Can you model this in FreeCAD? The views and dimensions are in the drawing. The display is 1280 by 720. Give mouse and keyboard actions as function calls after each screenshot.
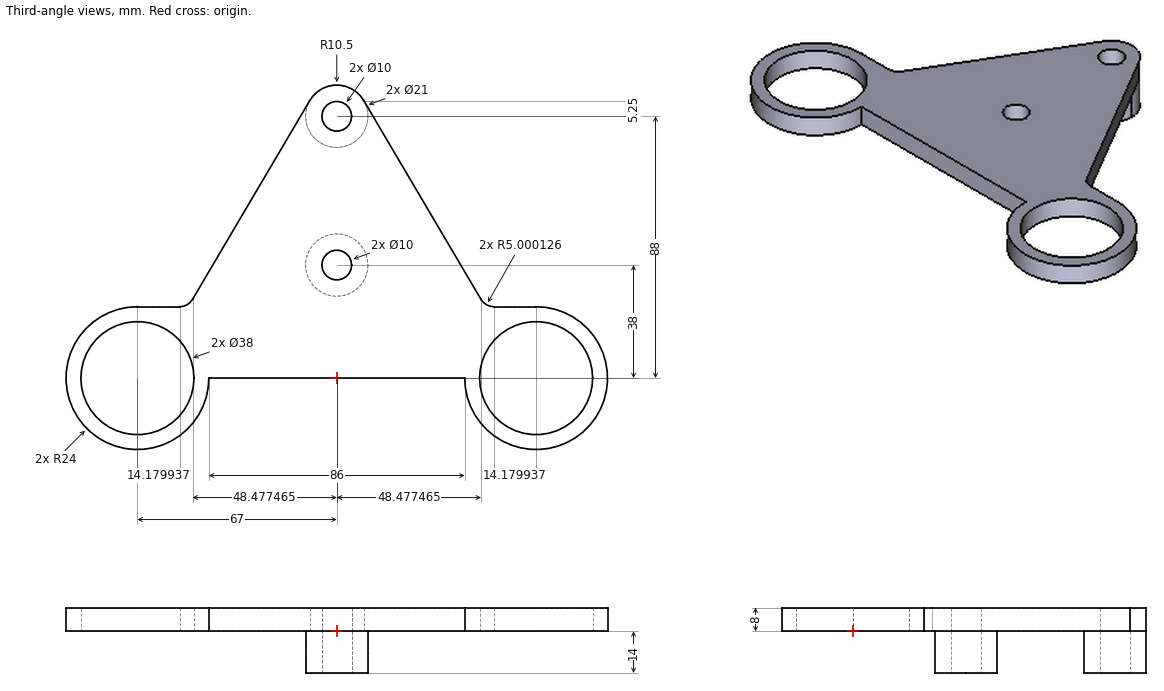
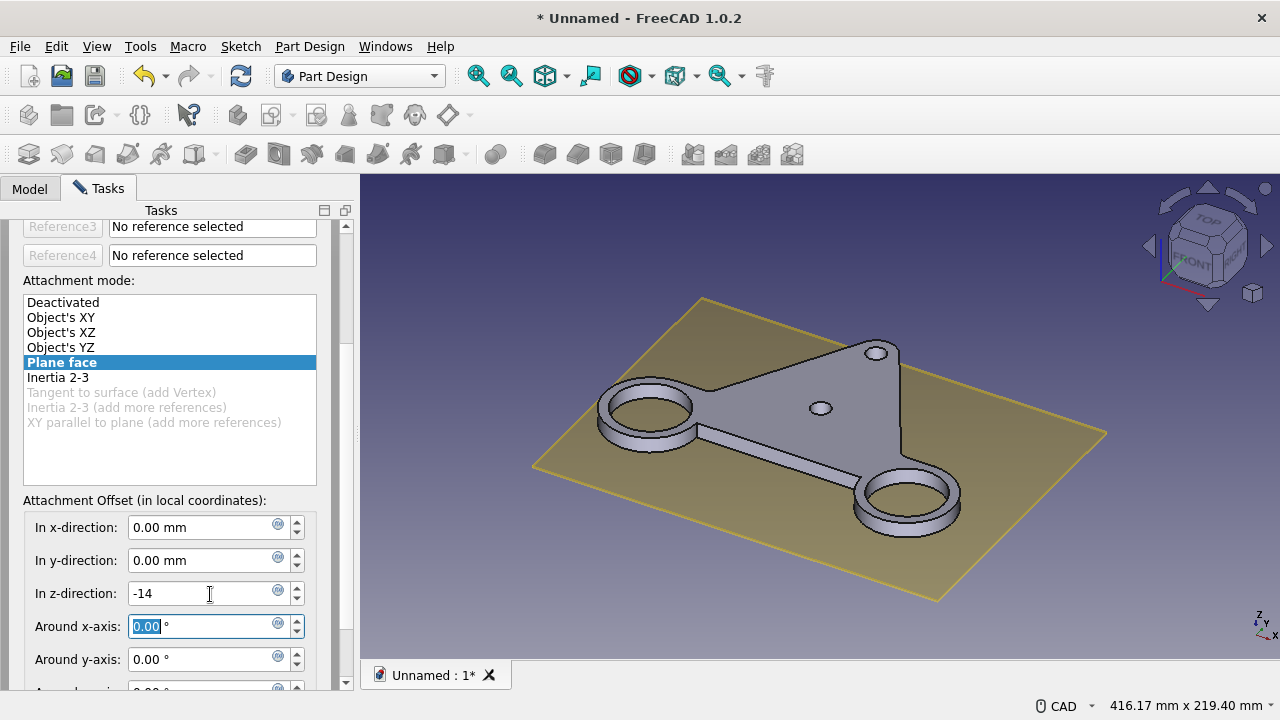
scroll(346, 455, up, 4)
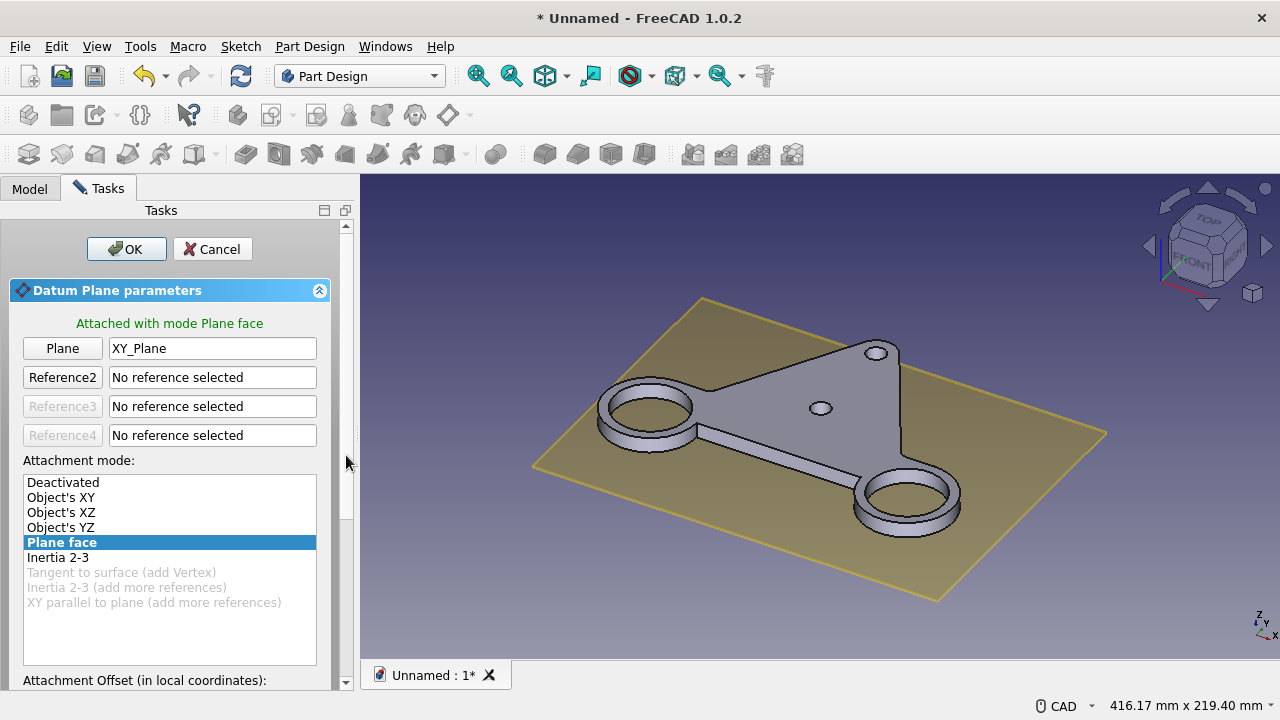
click(127, 249)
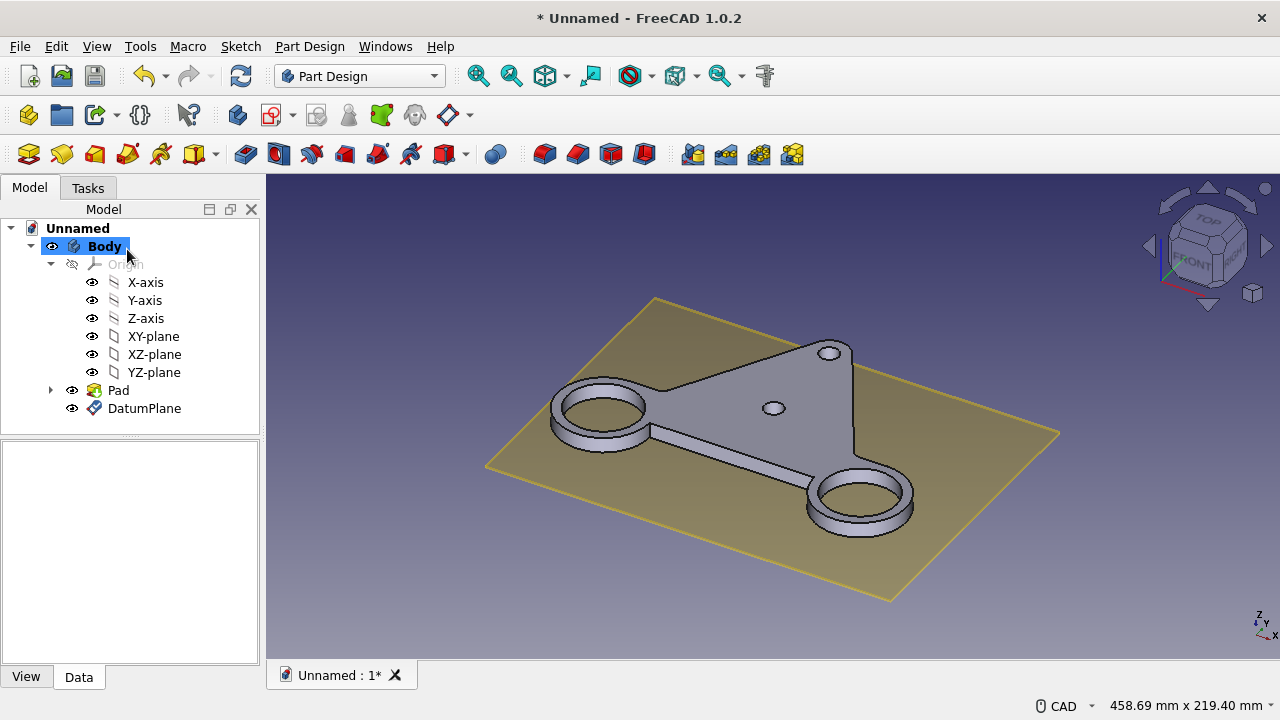
click(117, 408)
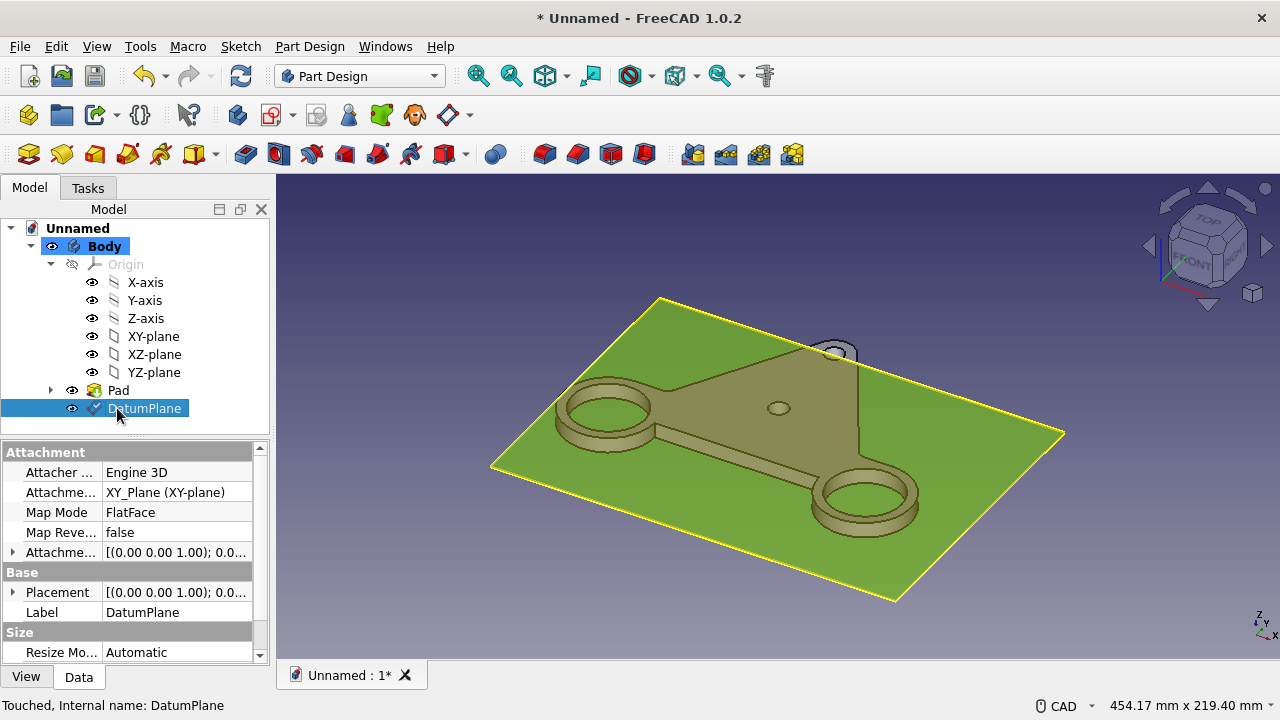
click(270, 116)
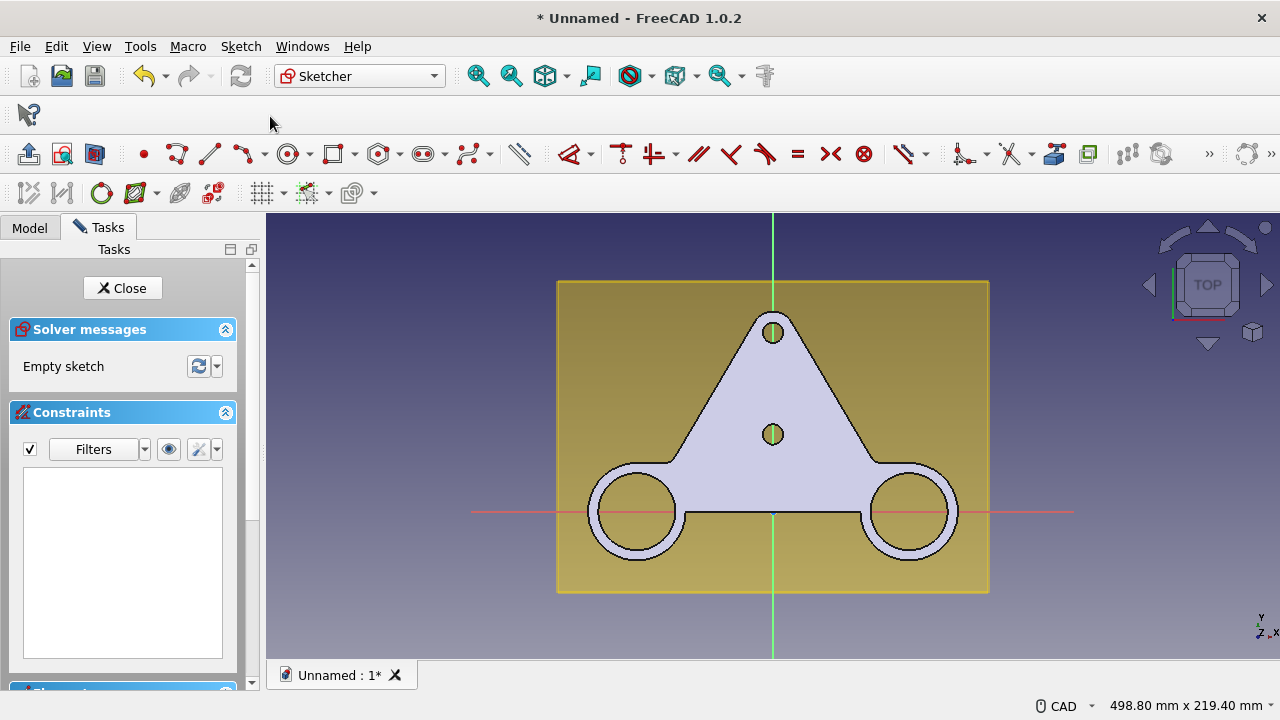
key(q)
key(s)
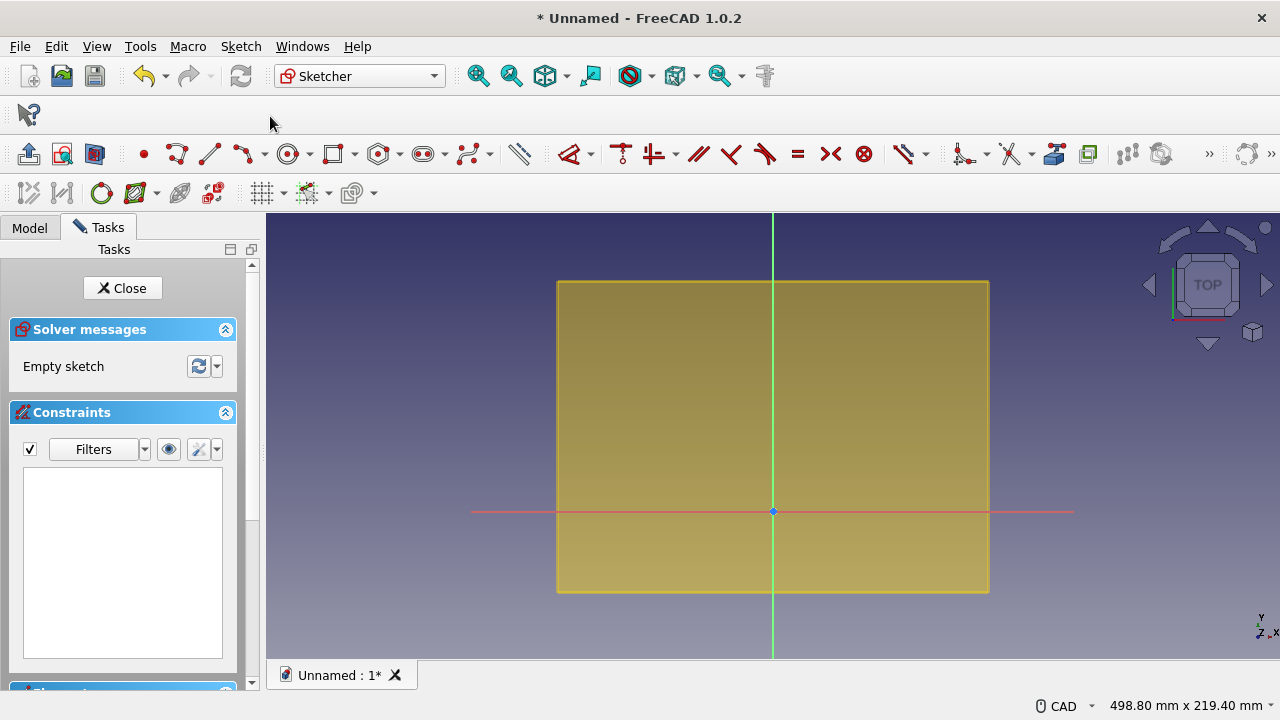
scroll(912, 362, up, 2)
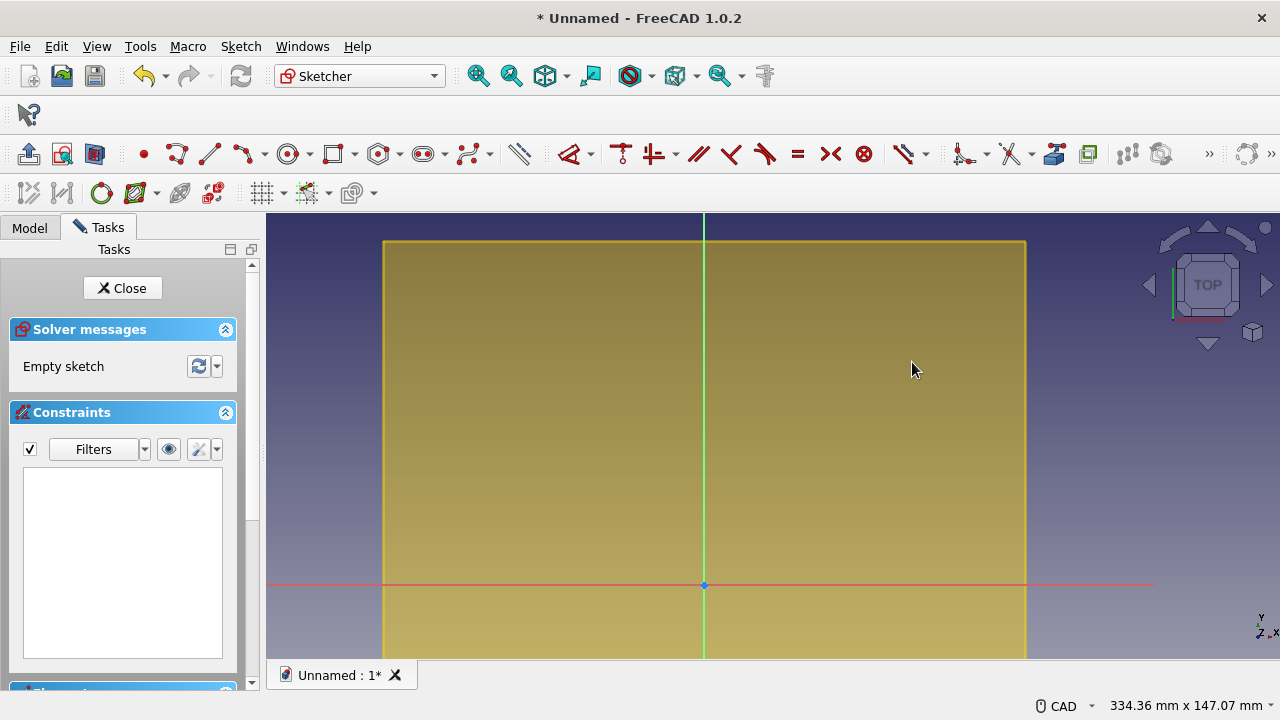
click(288, 154)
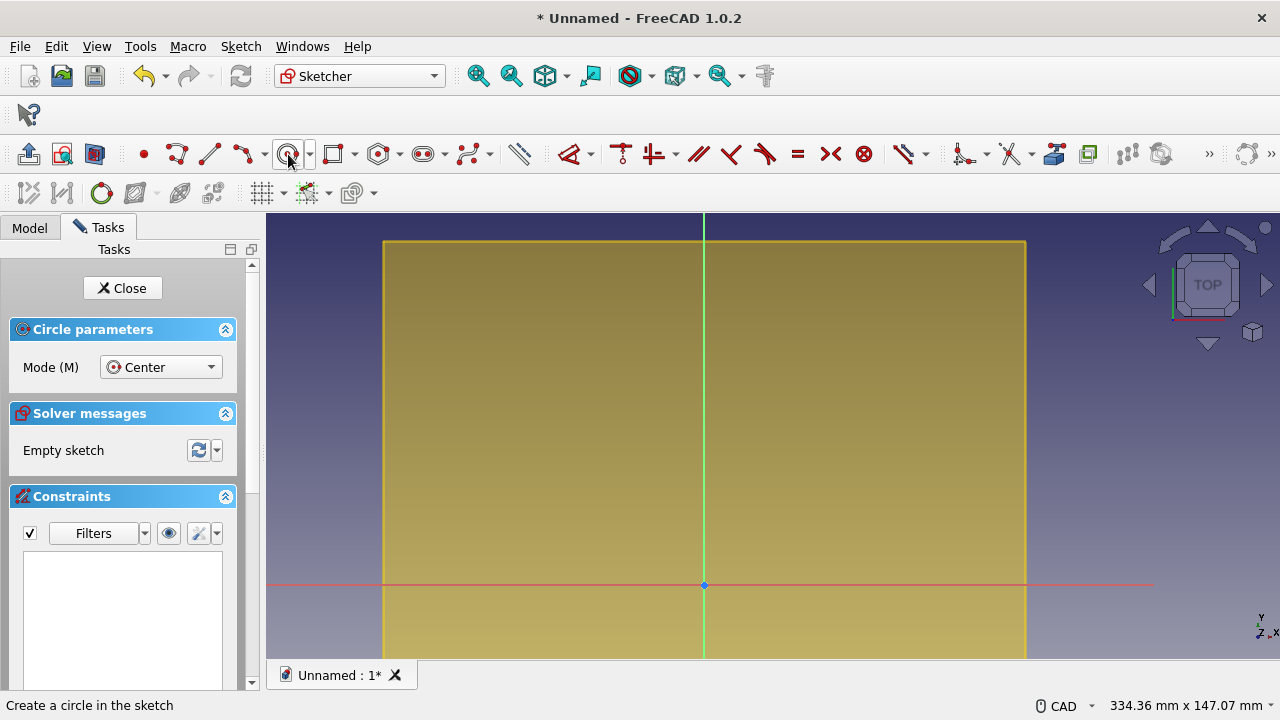
click(704, 318)
click(727, 296)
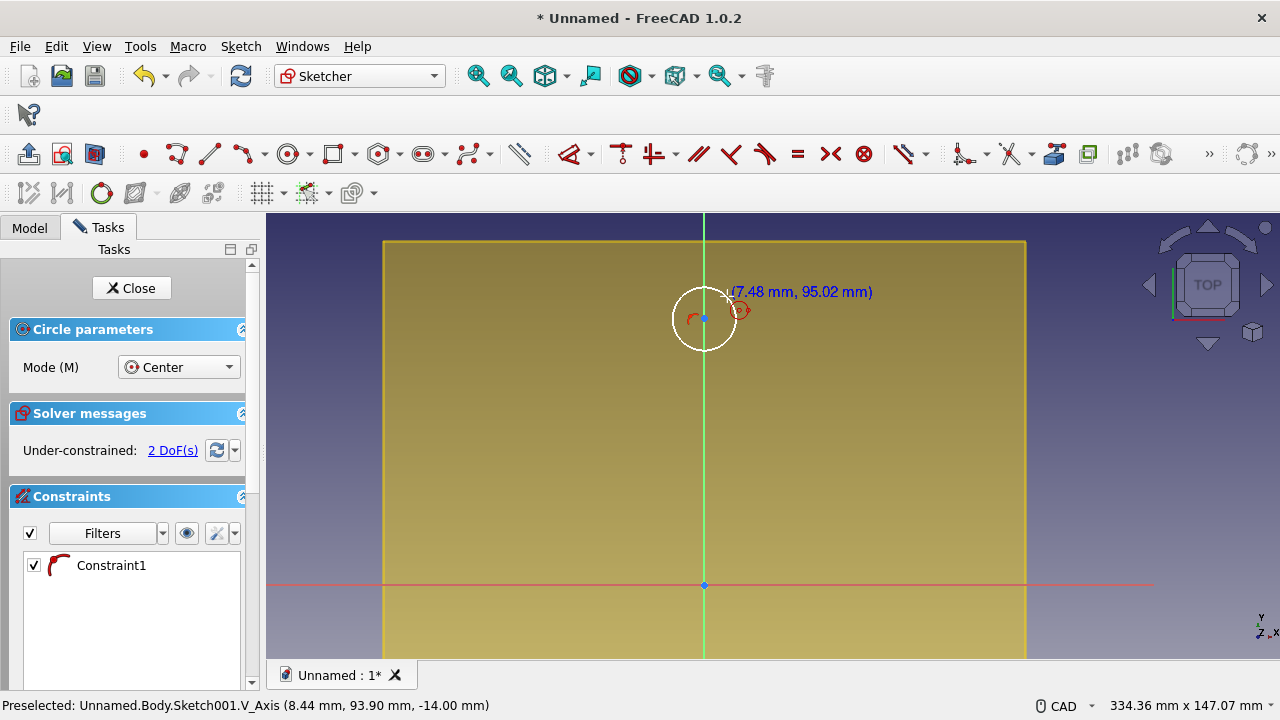
click(704, 470)
click(727, 447)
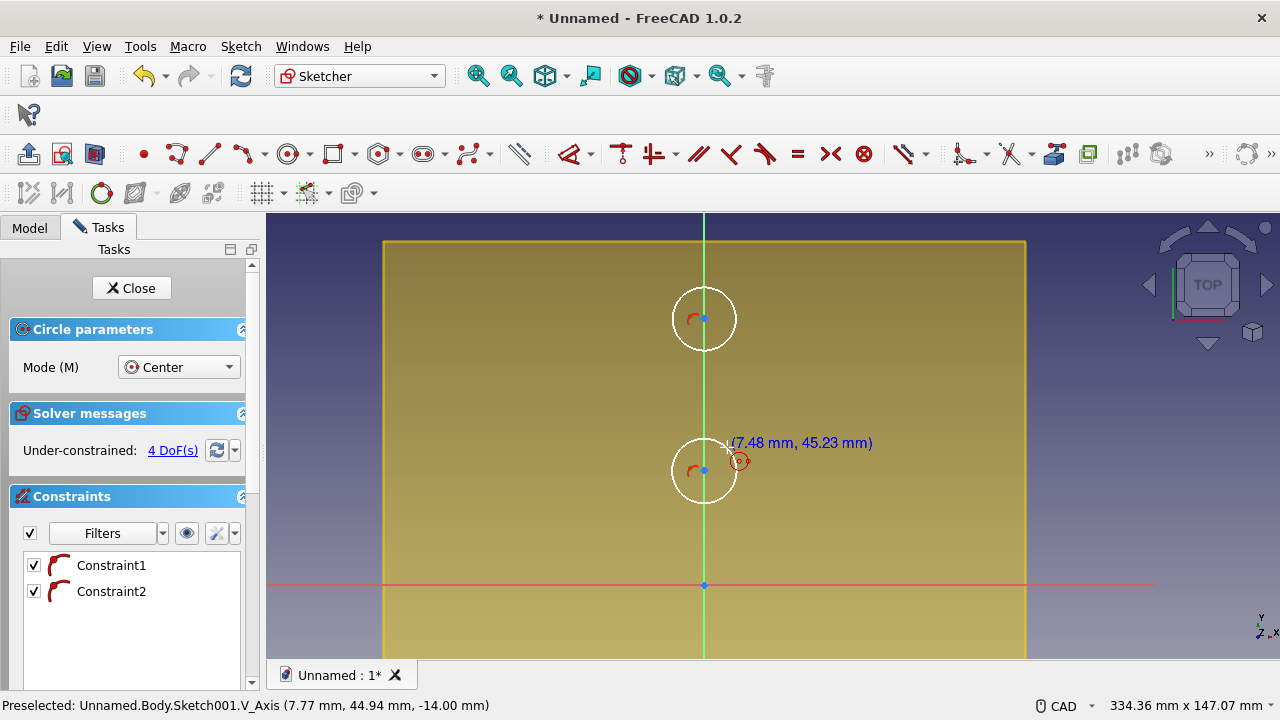
scroll(704, 318, up, 3)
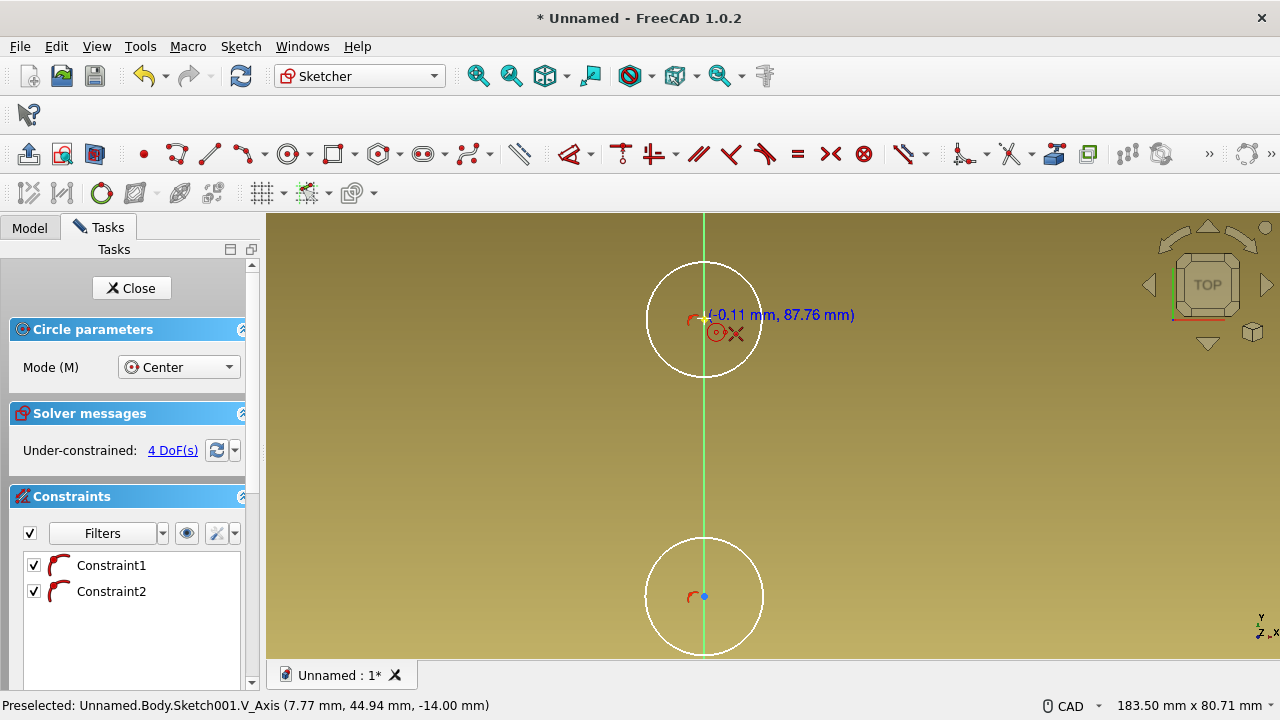
click(704, 320)
click(724, 299)